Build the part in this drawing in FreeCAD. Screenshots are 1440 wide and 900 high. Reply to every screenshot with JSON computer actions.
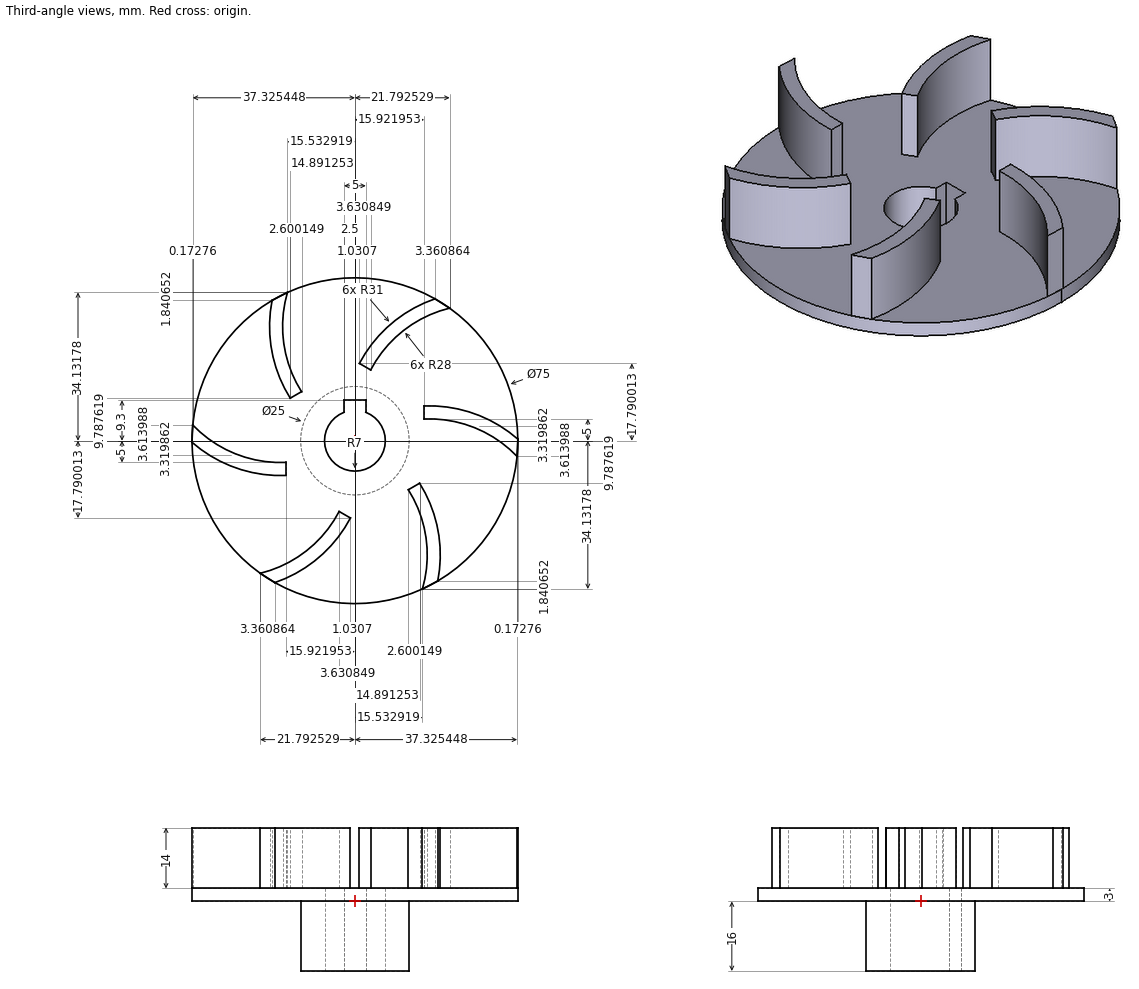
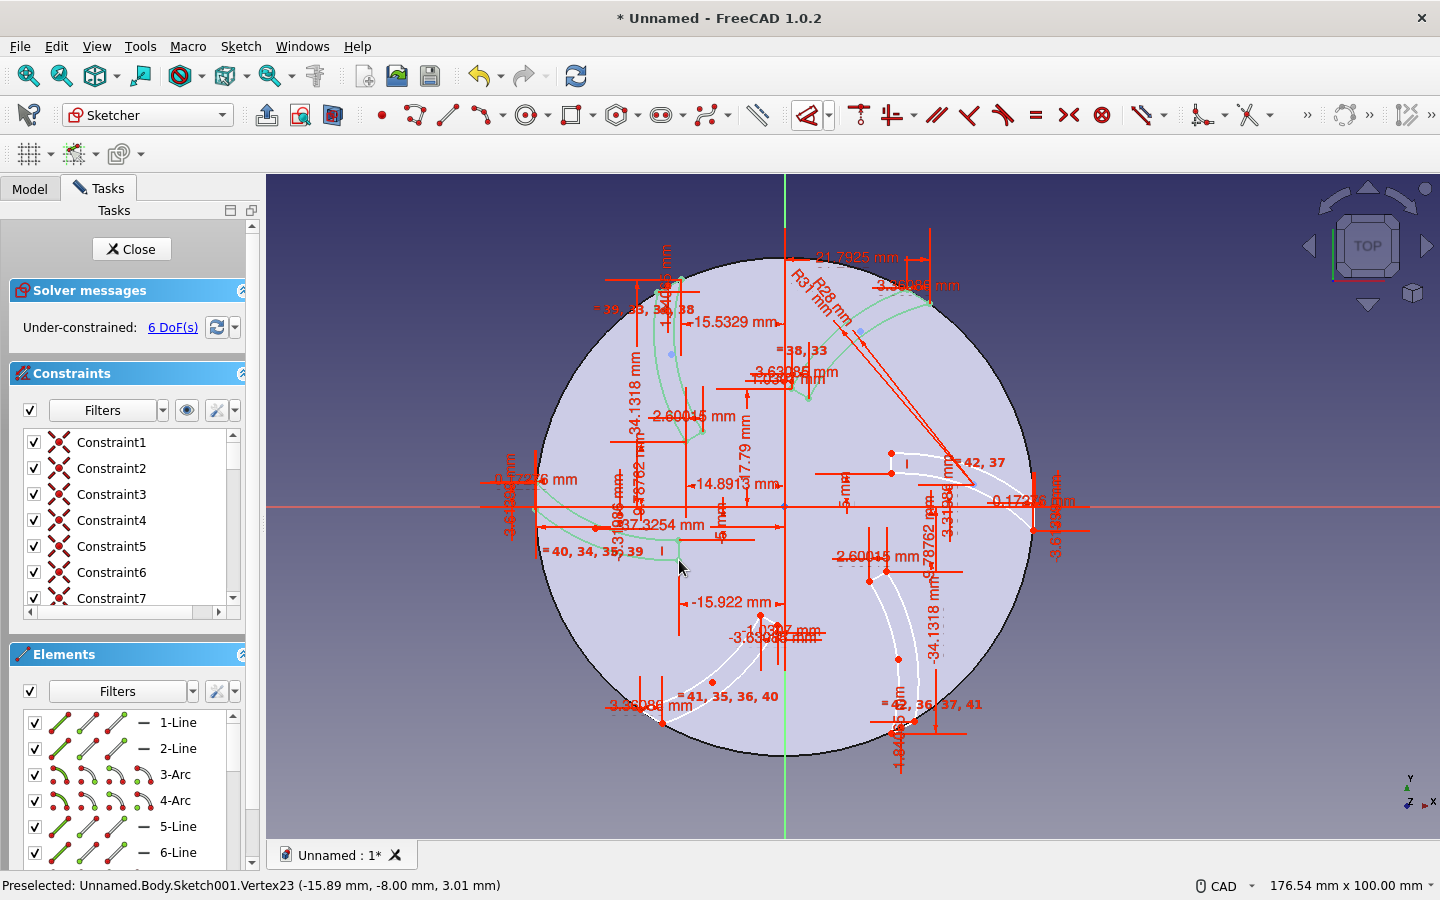
{"action": "left_click", "coordinate": [640, 710]}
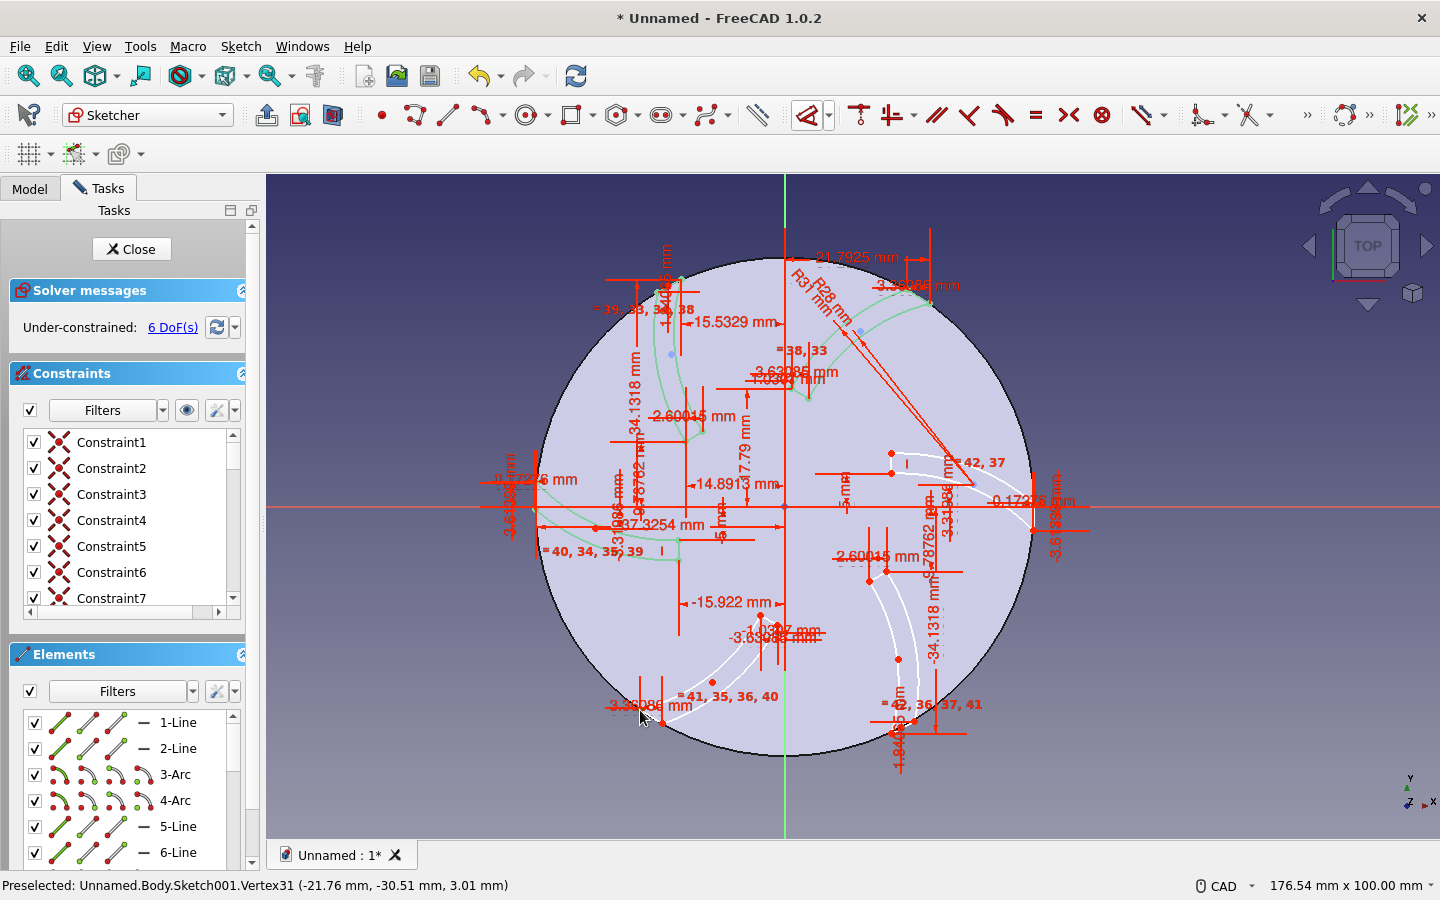
{"action": "key", "text": "l"}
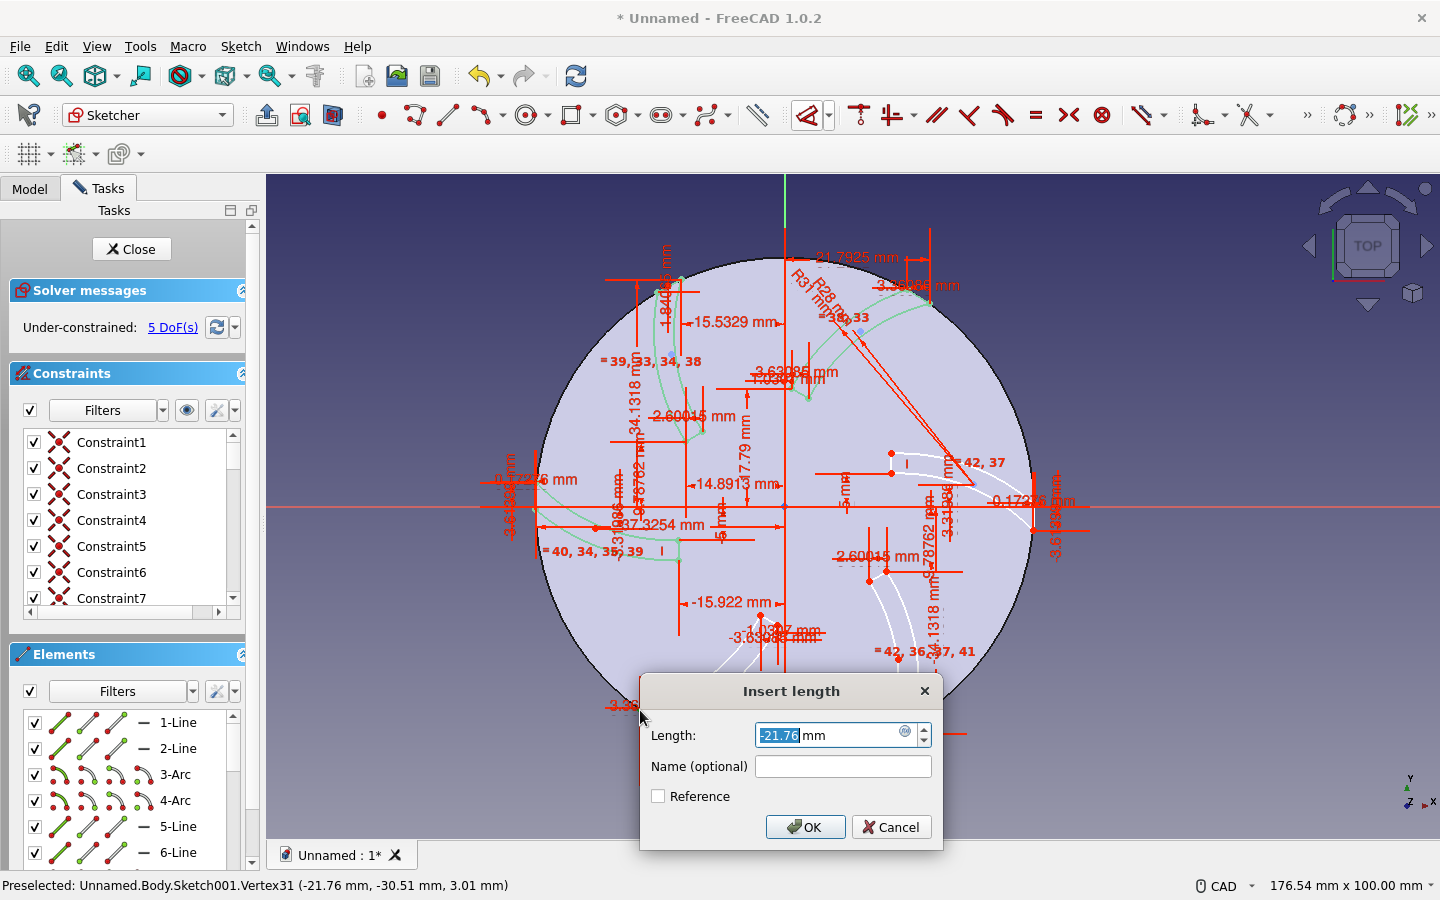
{"action": "type", "text": "-21.792529"}
{"action": "key", "text": "Return"}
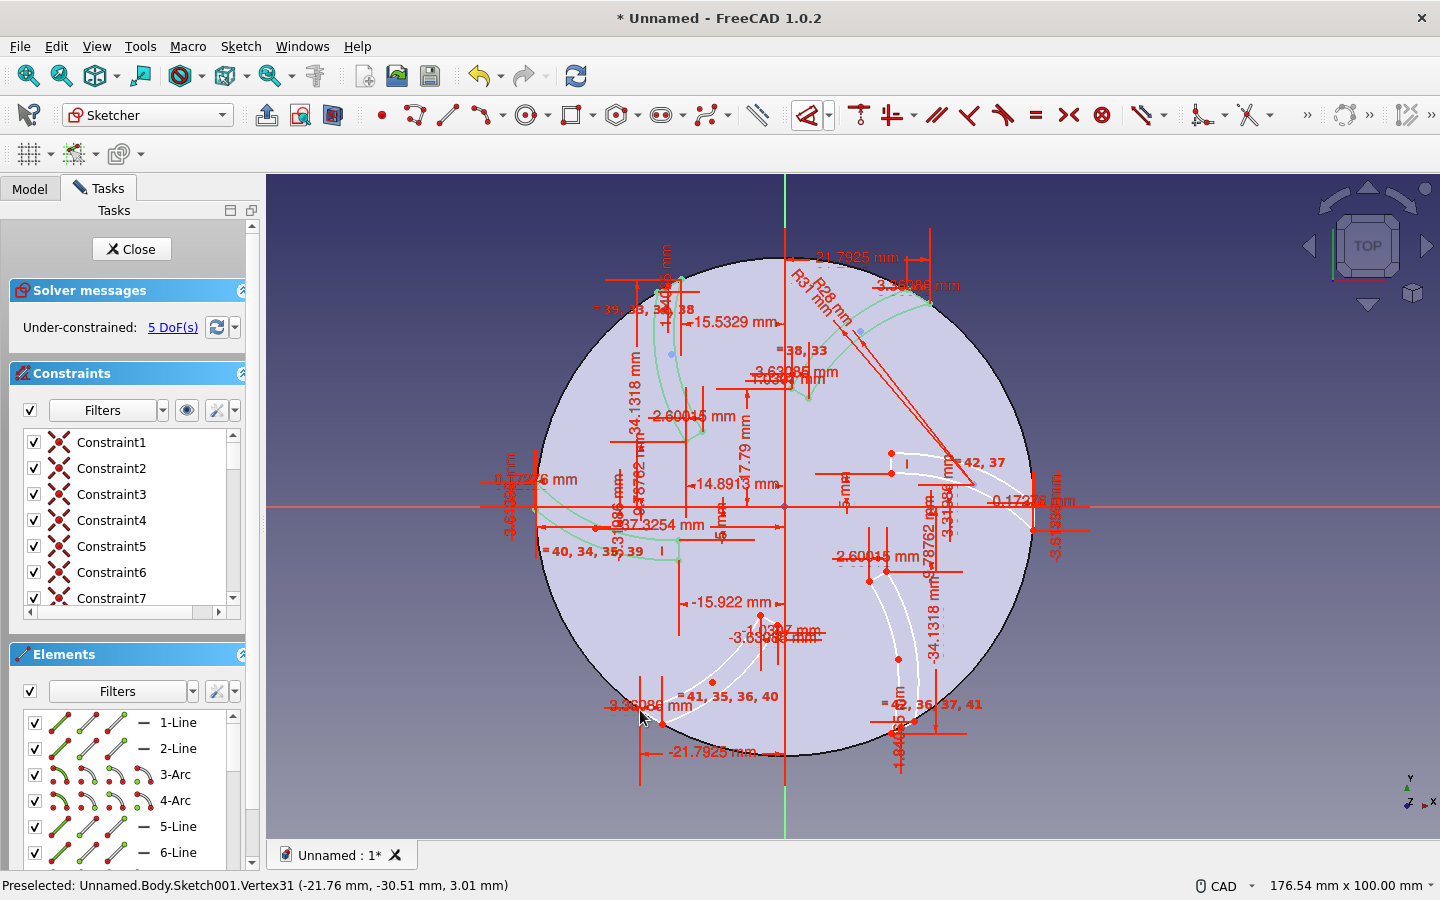
{"action": "left_click", "coordinate": [778, 625]}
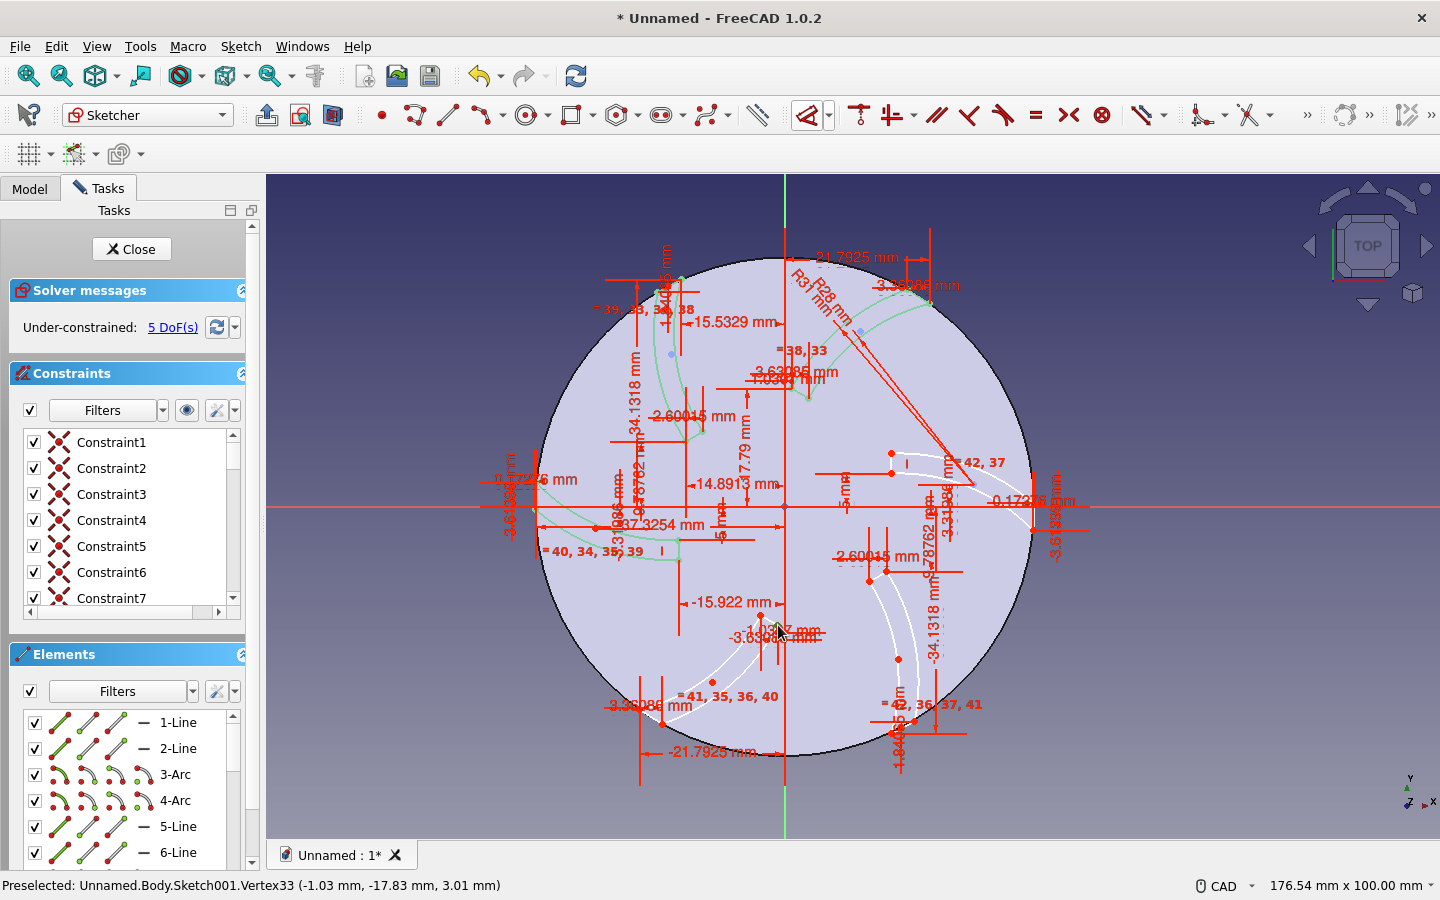
{"action": "key", "text": "i"}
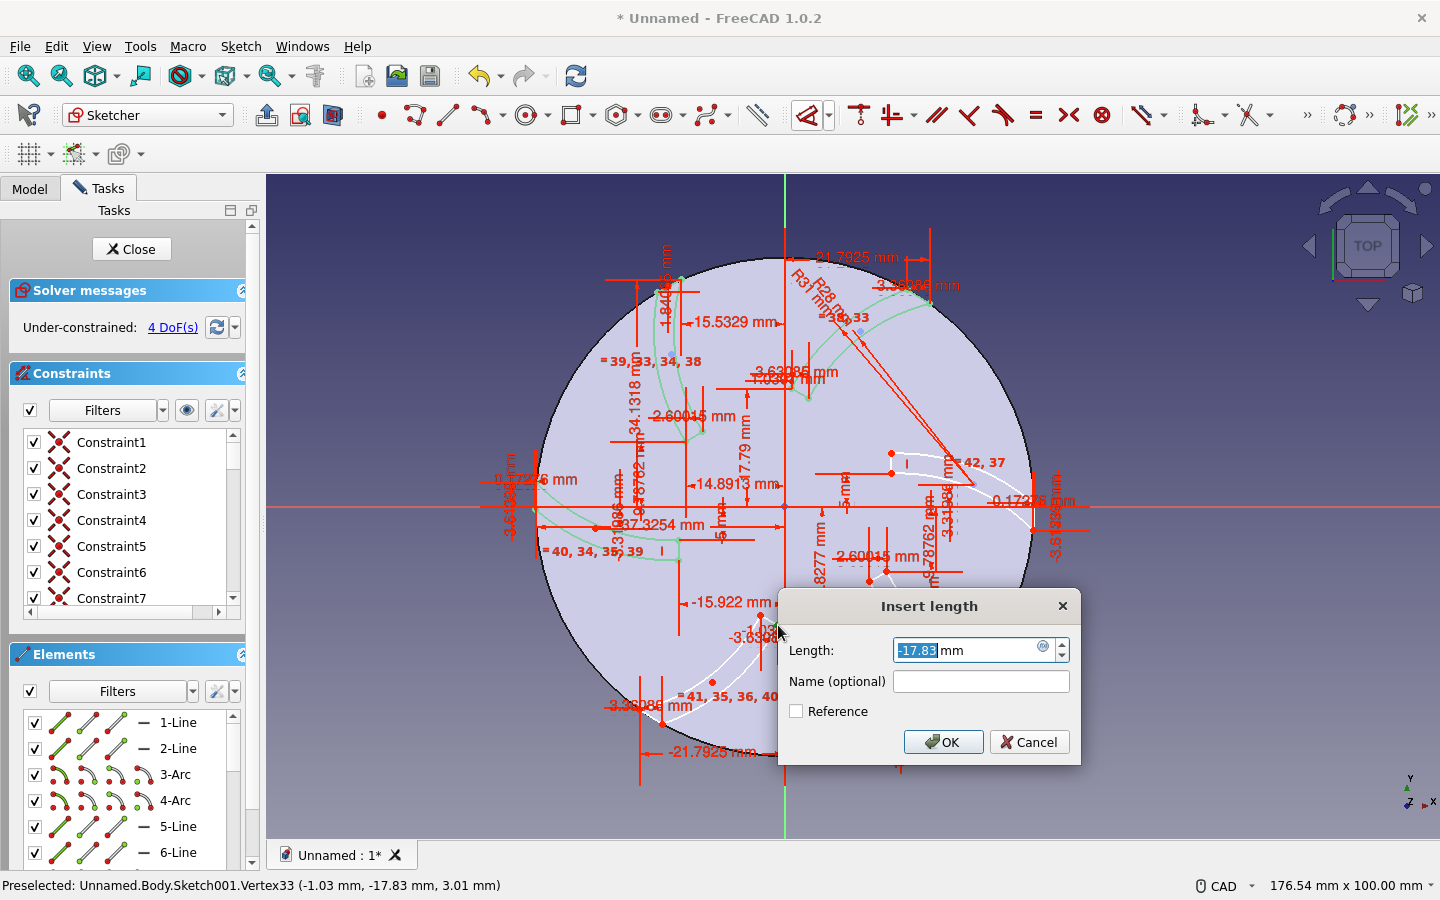
{"action": "type", "text": "-17.790013"}
{"action": "key", "text": "Return"}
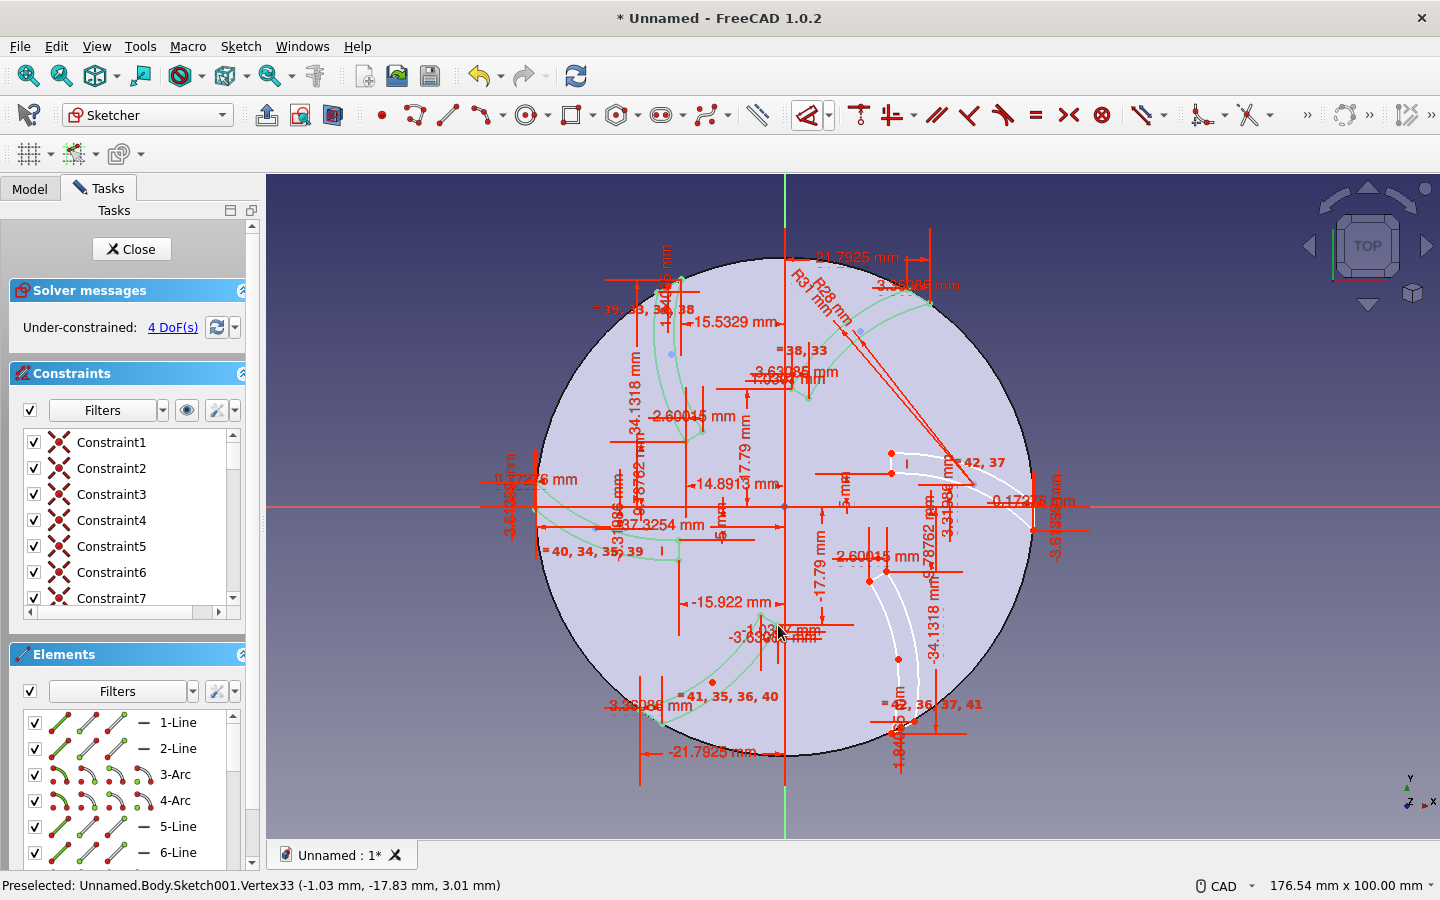
{"action": "left_click", "coordinate": [891, 734]}